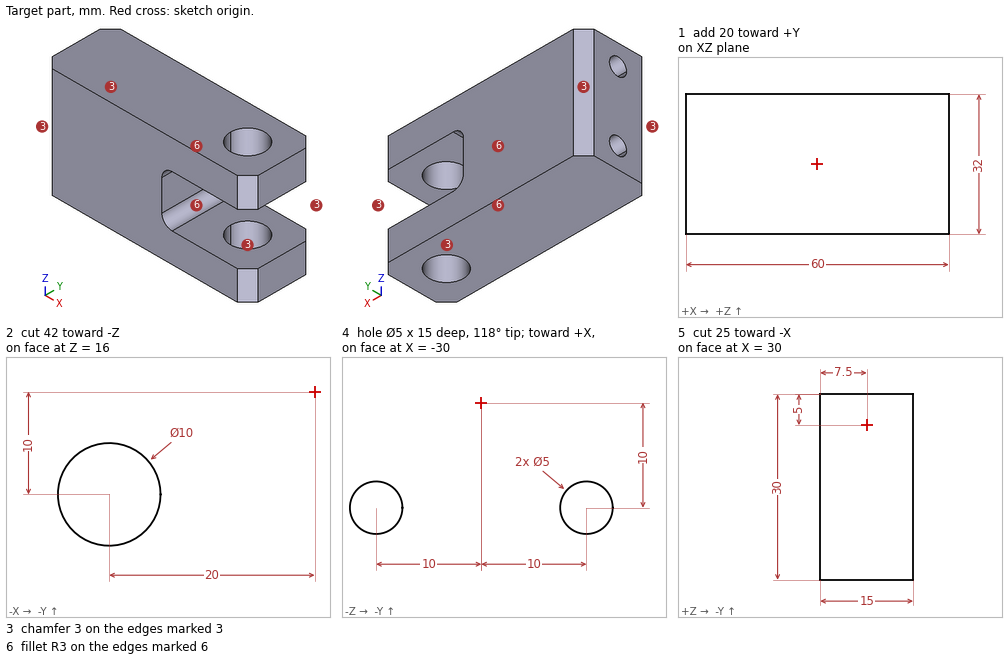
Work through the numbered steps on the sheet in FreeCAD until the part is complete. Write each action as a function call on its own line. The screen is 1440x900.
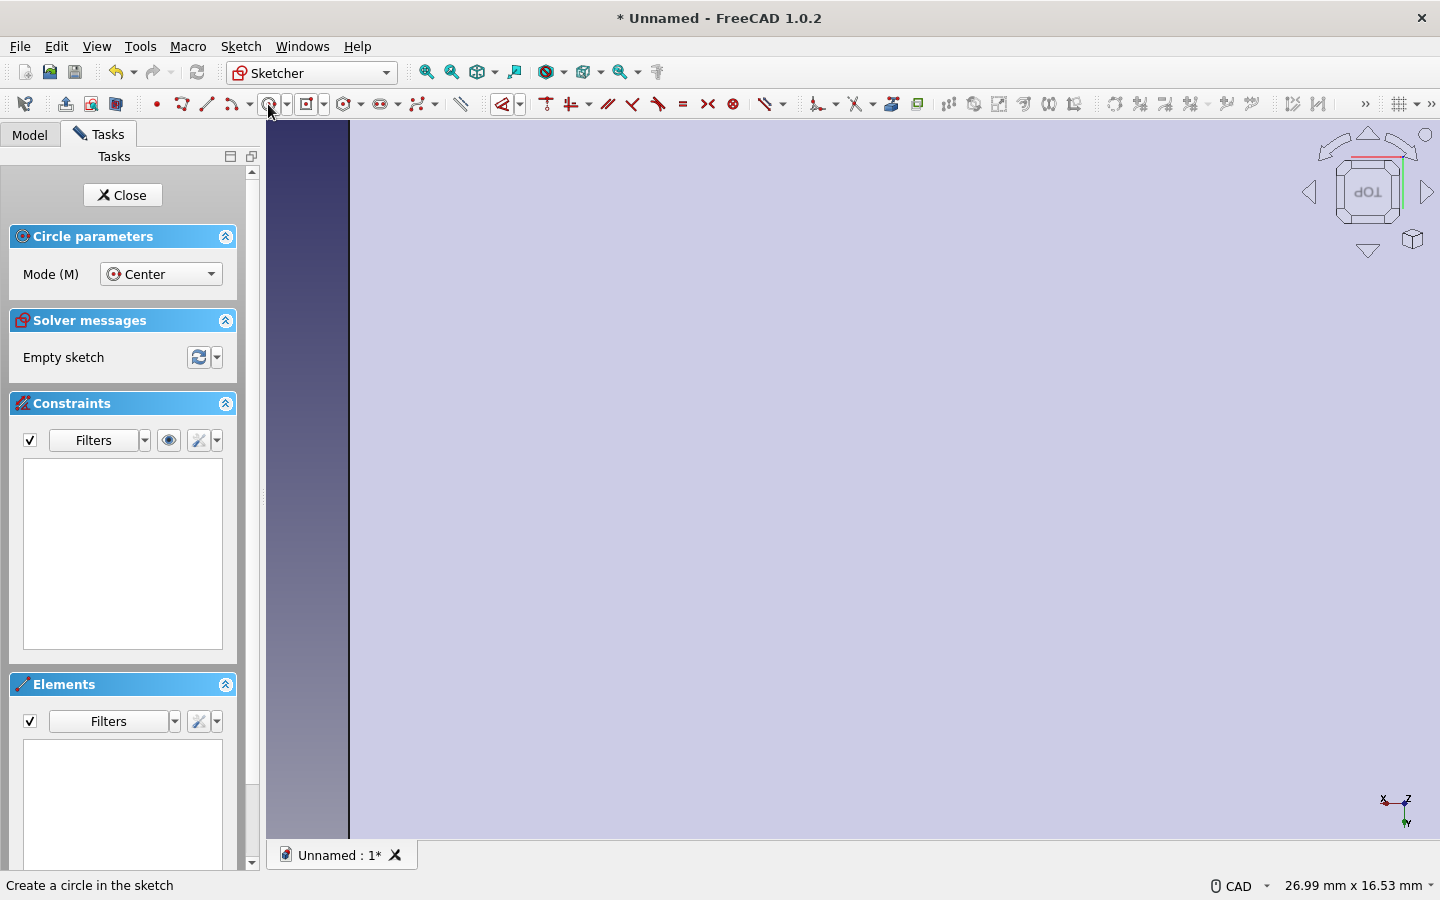
click(784, 475)
click(938, 321)
key(Escape)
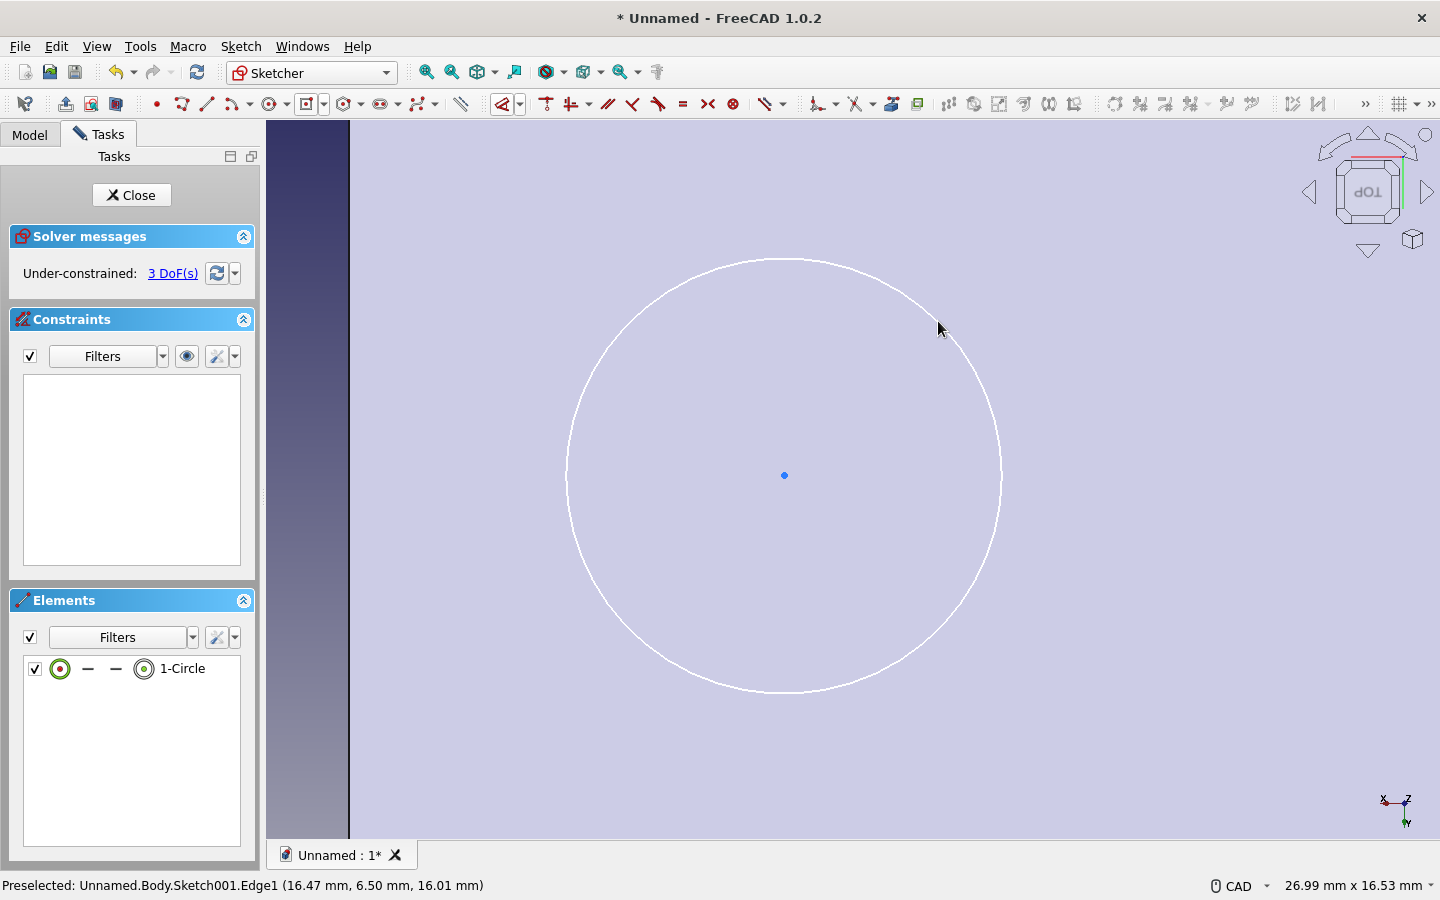
click(938, 322)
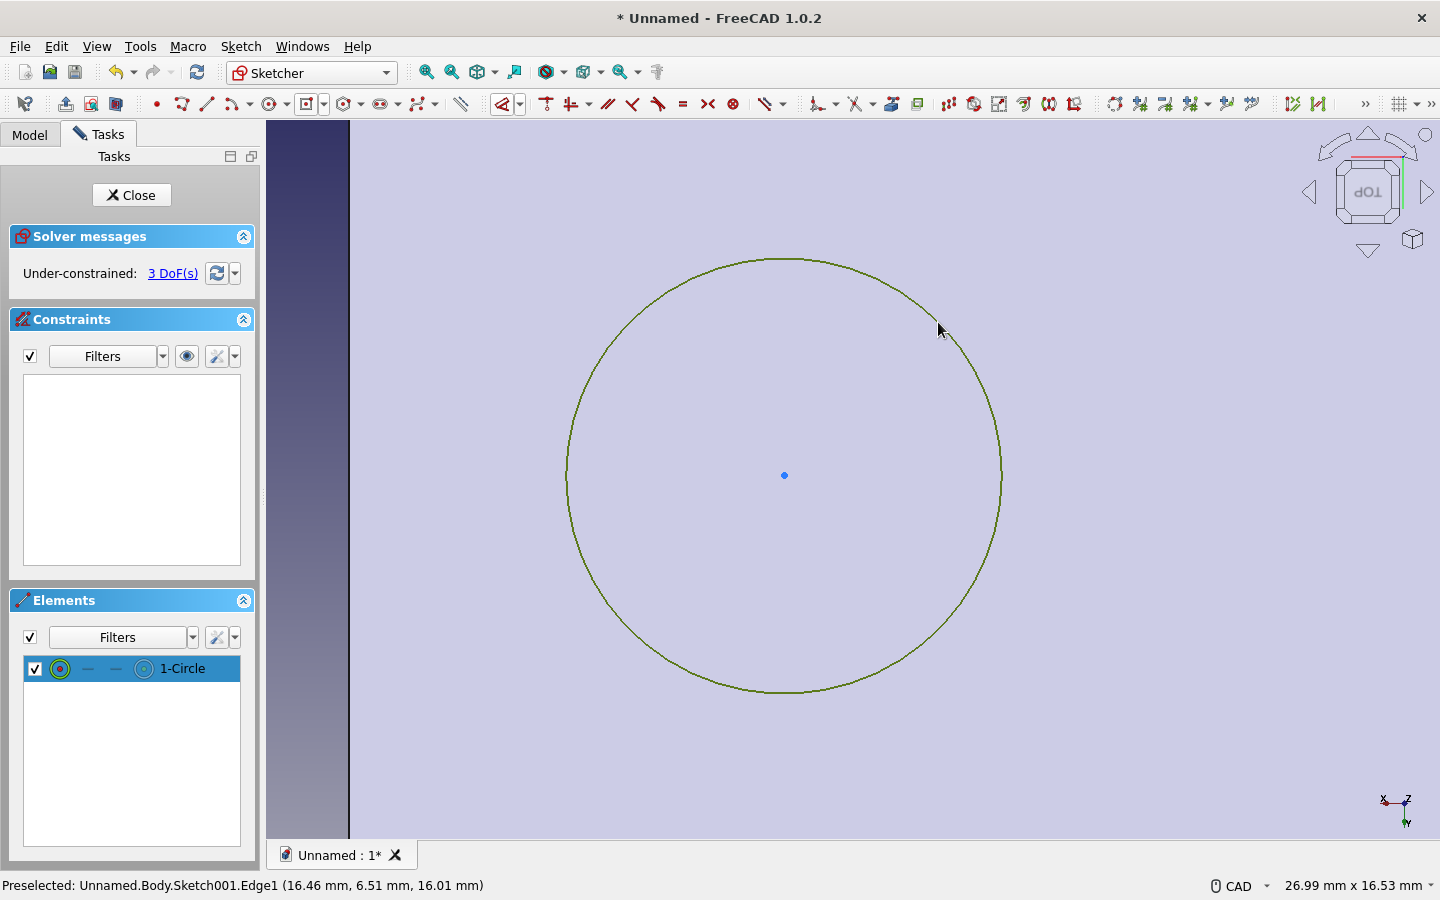
click(520, 104)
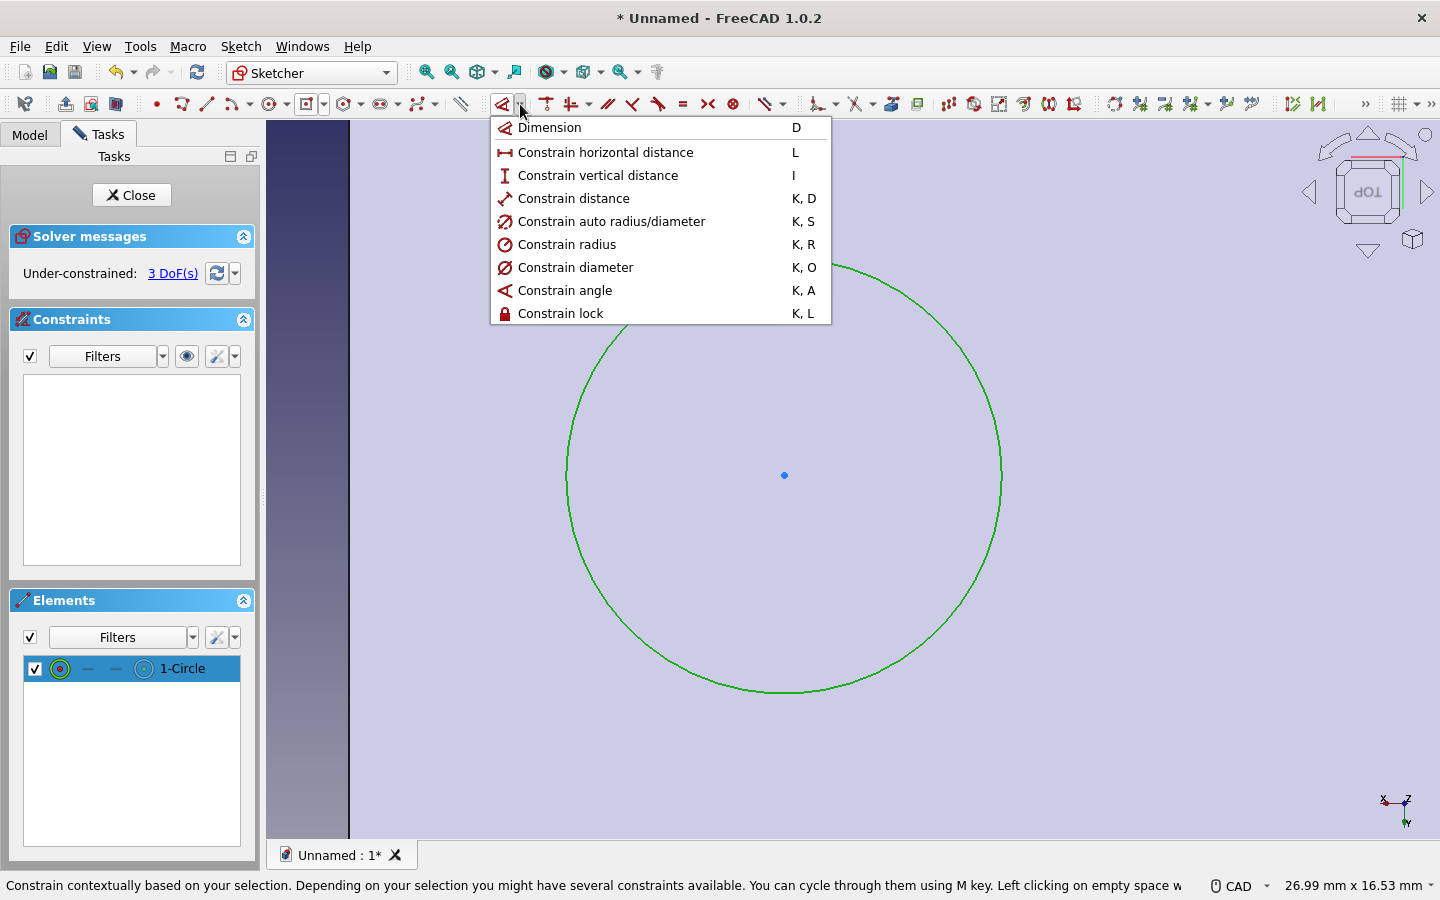
click(661, 268)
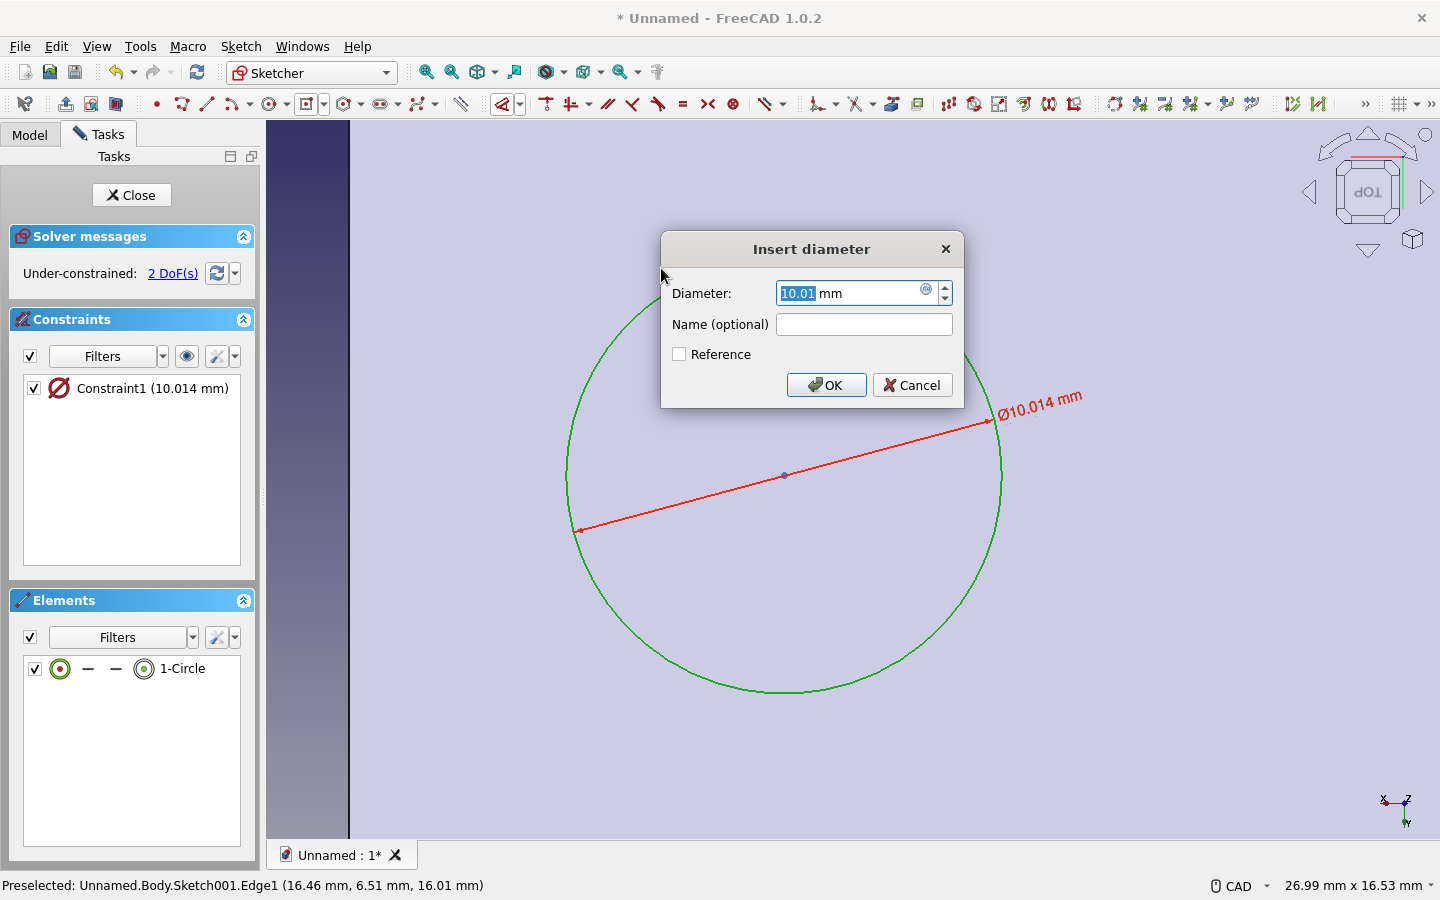
text(10)
key(Return)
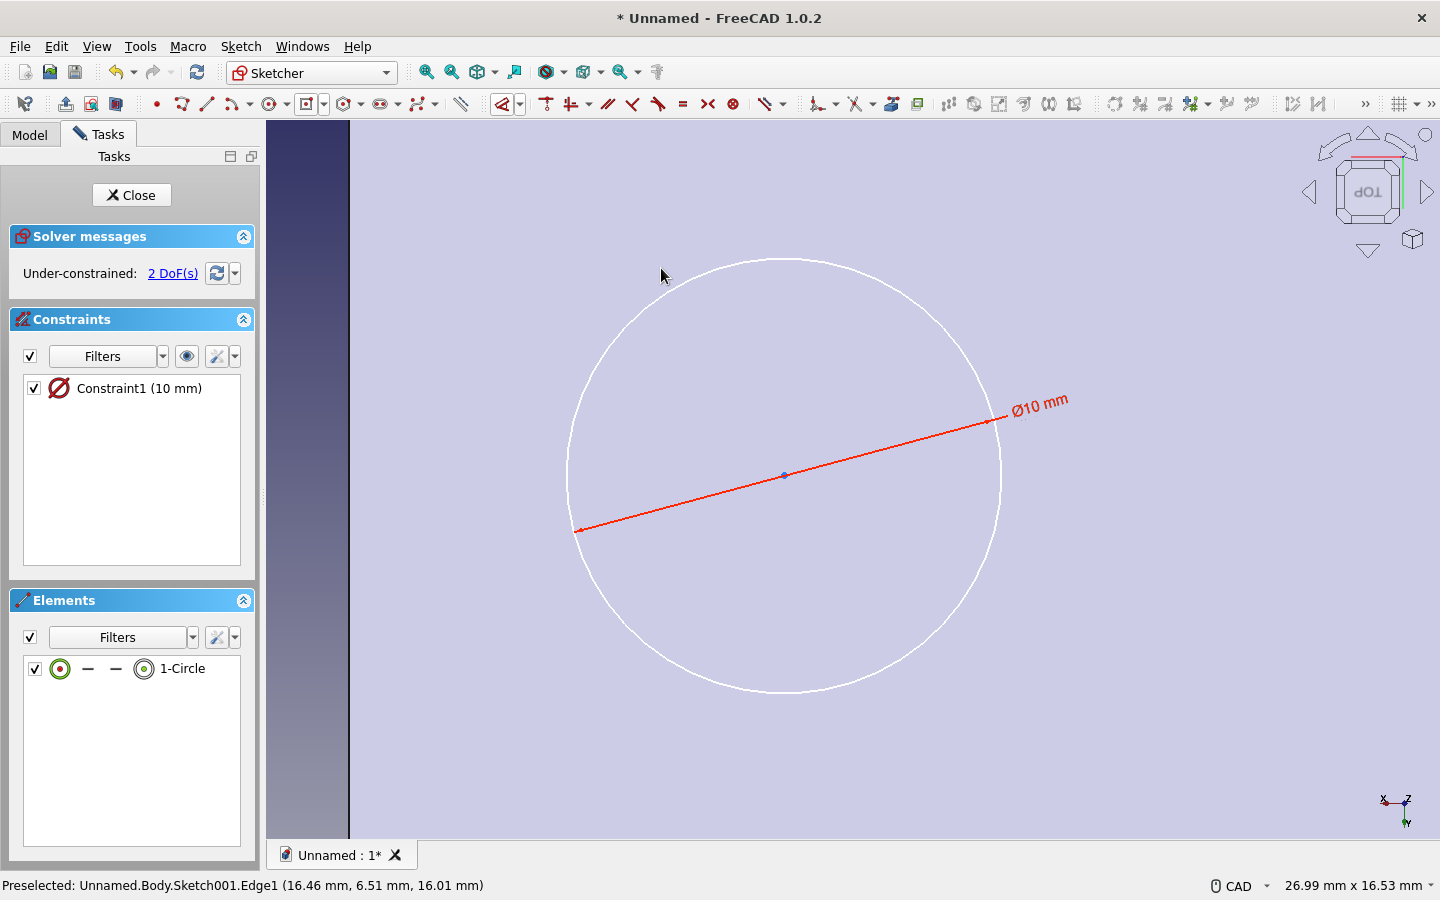
click(784, 476)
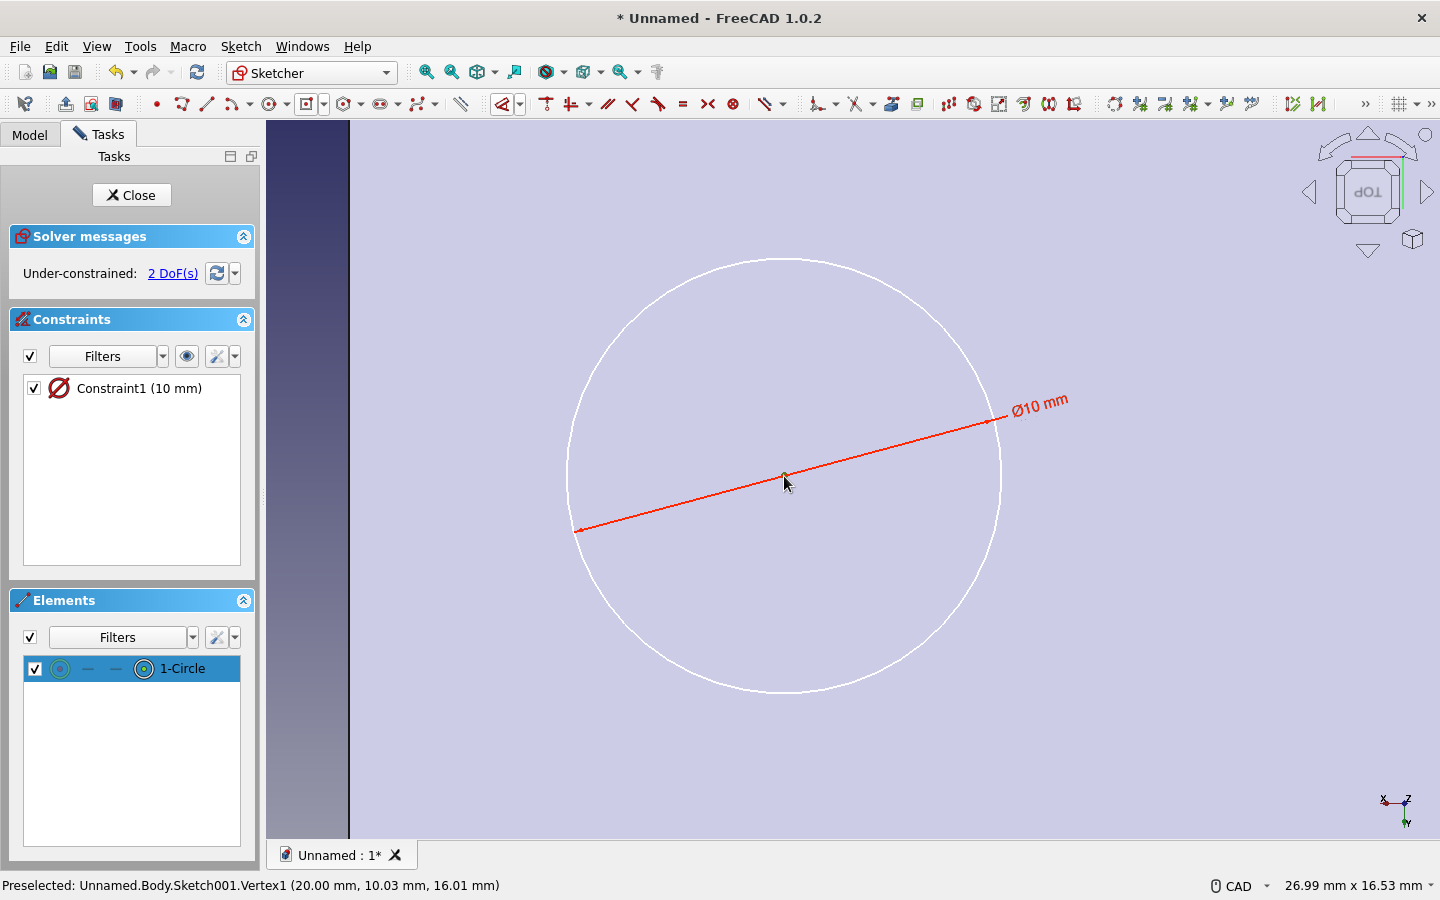
click(520, 104)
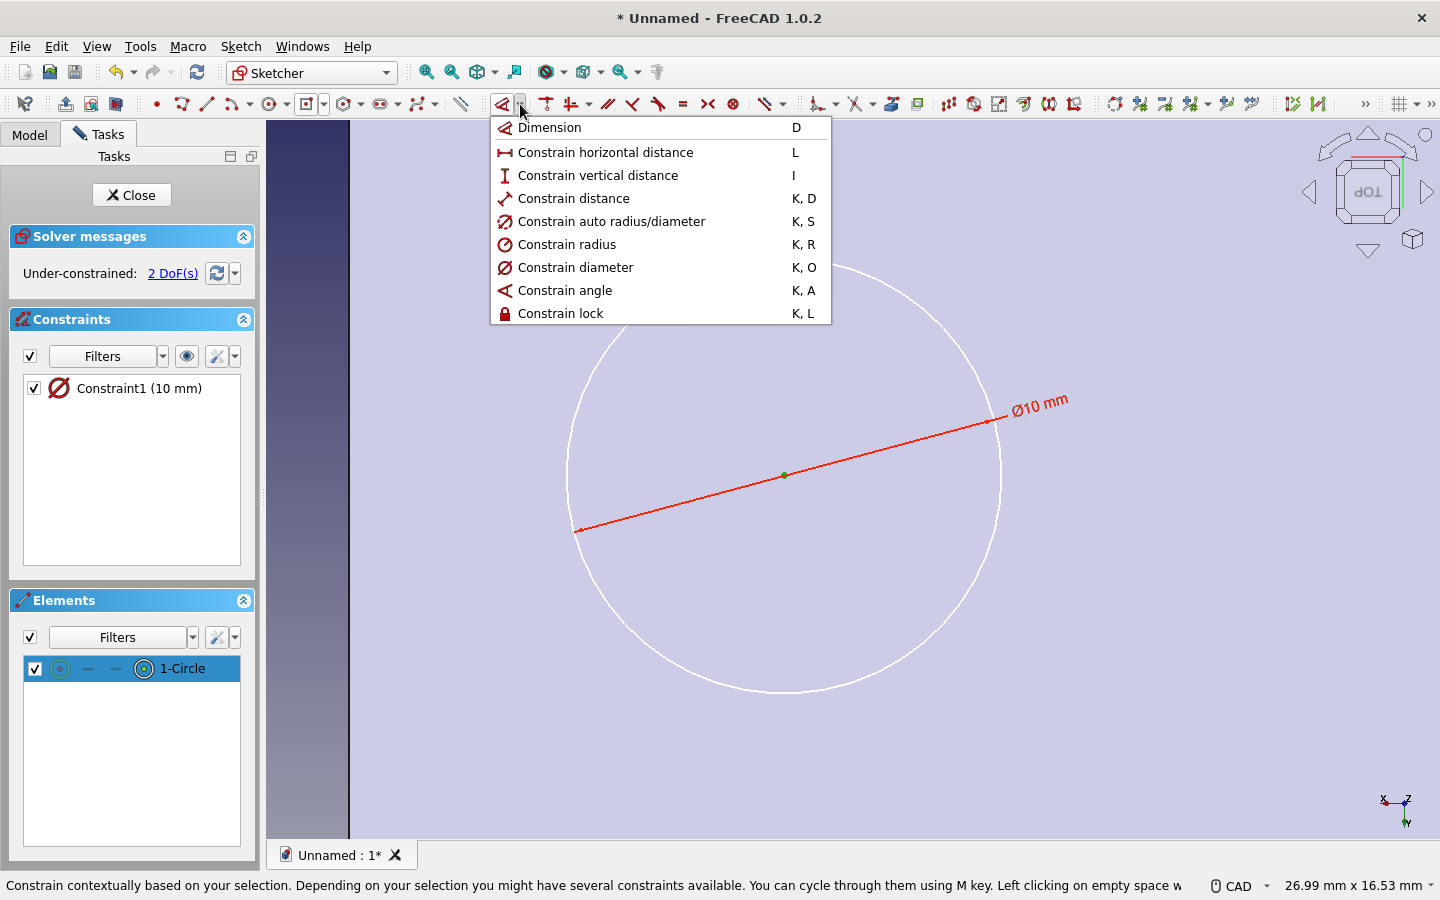
click(661, 152)